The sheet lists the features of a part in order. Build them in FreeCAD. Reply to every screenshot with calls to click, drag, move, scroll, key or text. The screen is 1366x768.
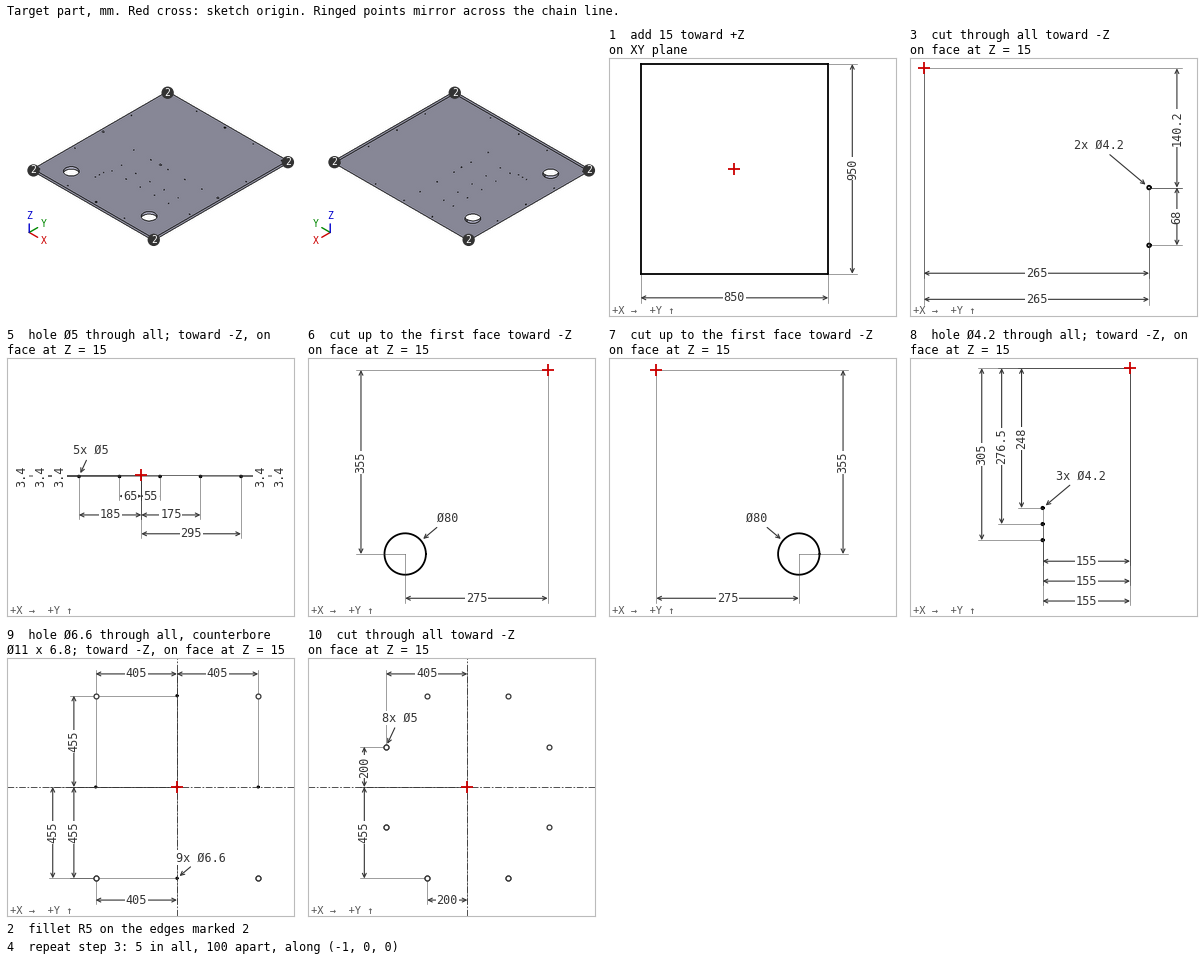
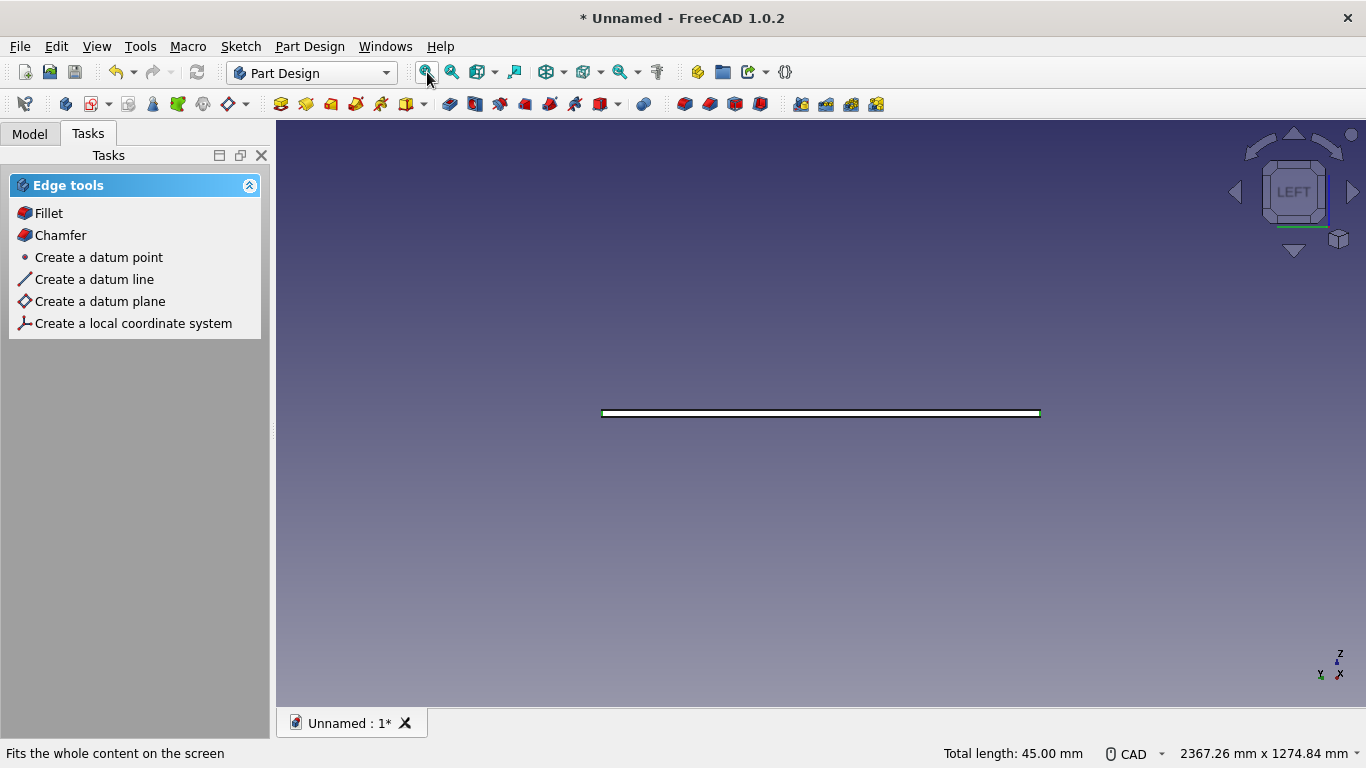
key(0)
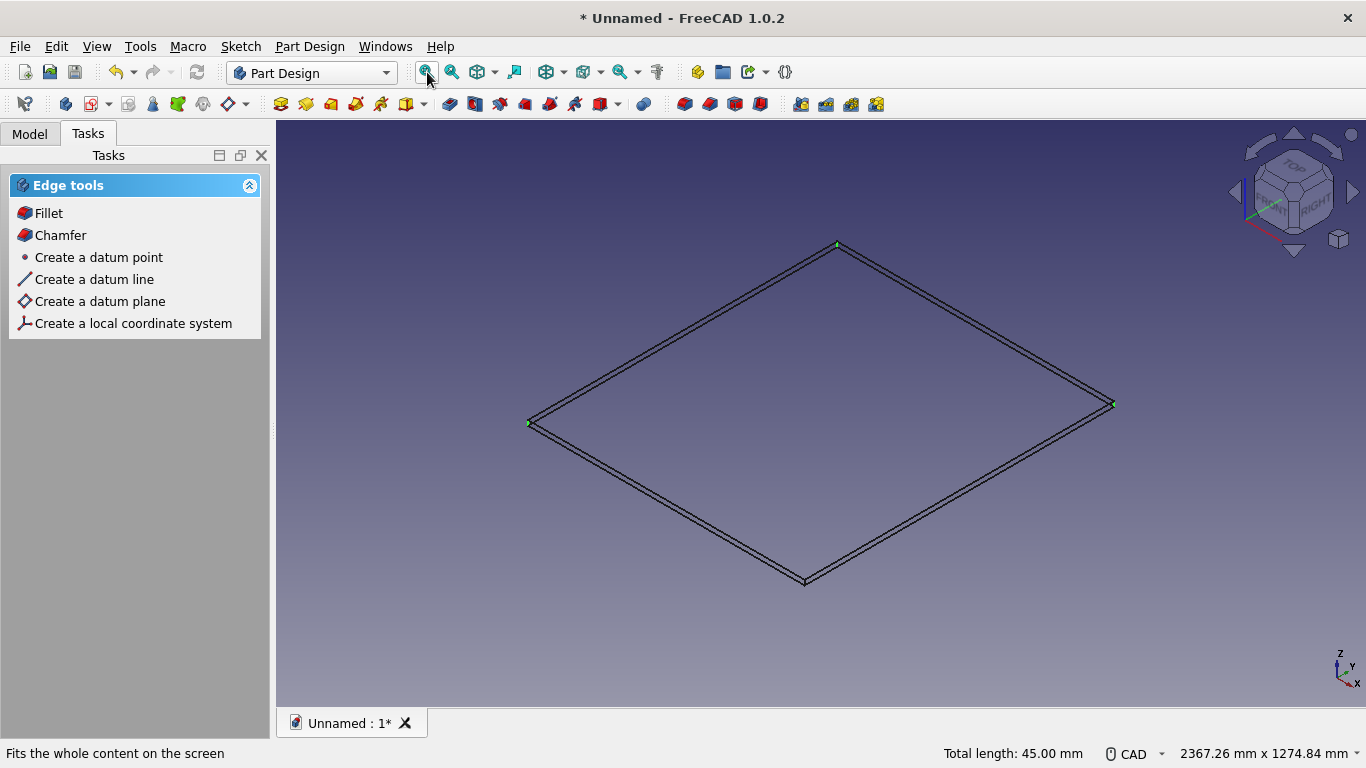
scroll(805, 582, up, 9)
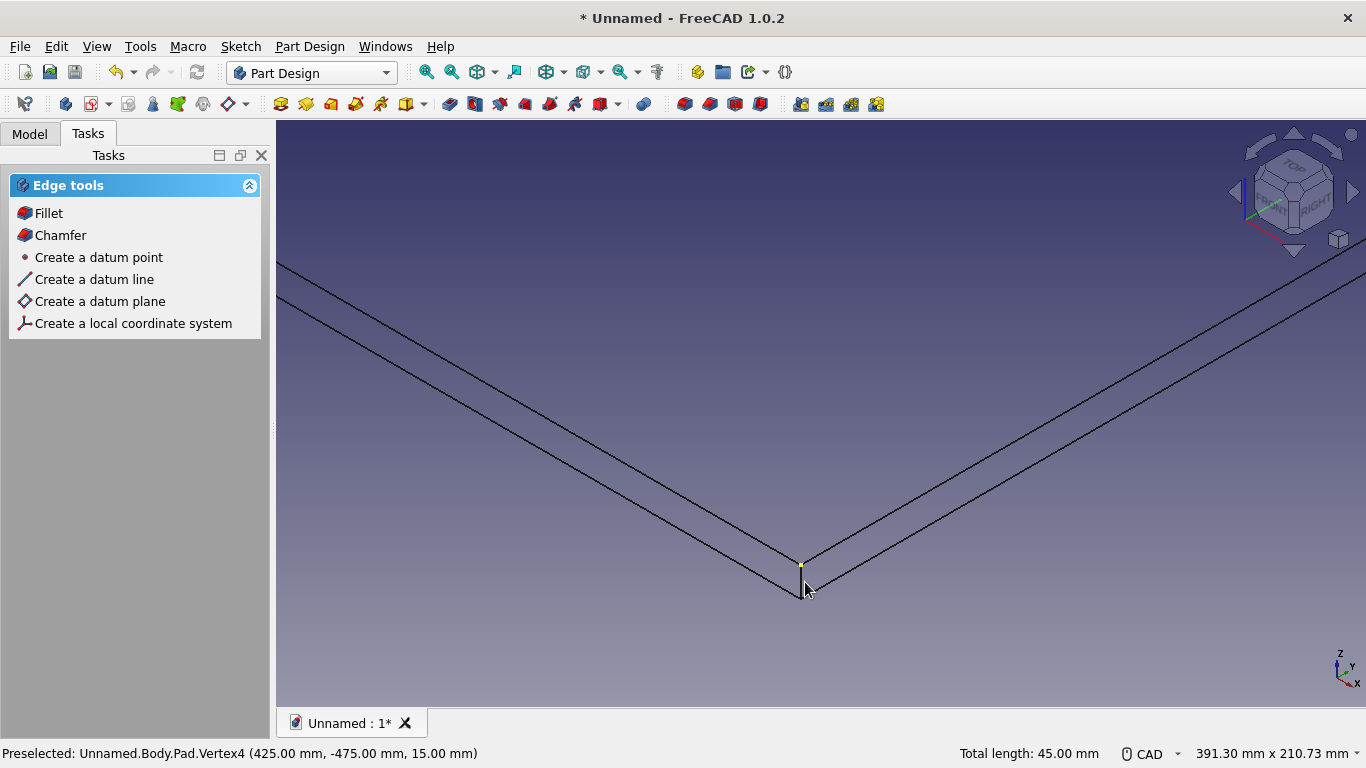
click(801, 581, ctrl)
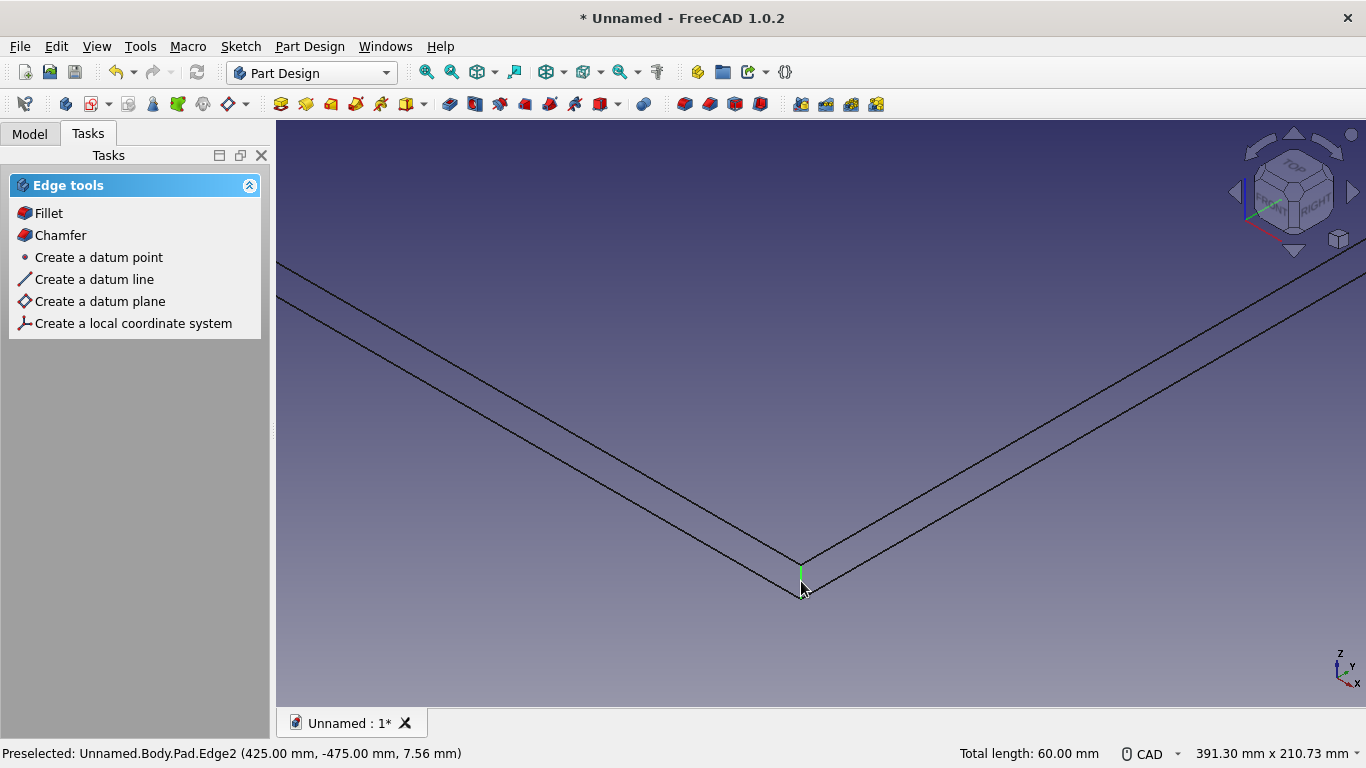
key(v)
key(1)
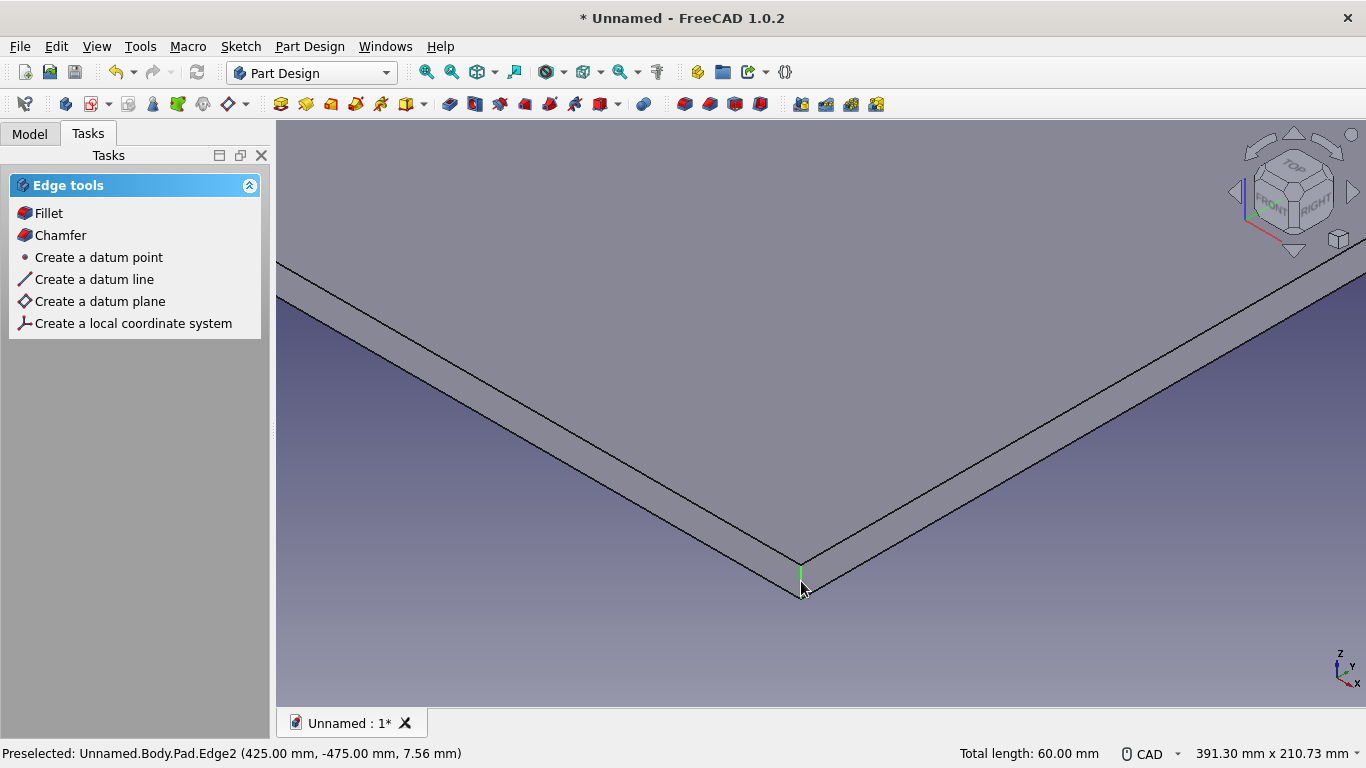
click(685, 104)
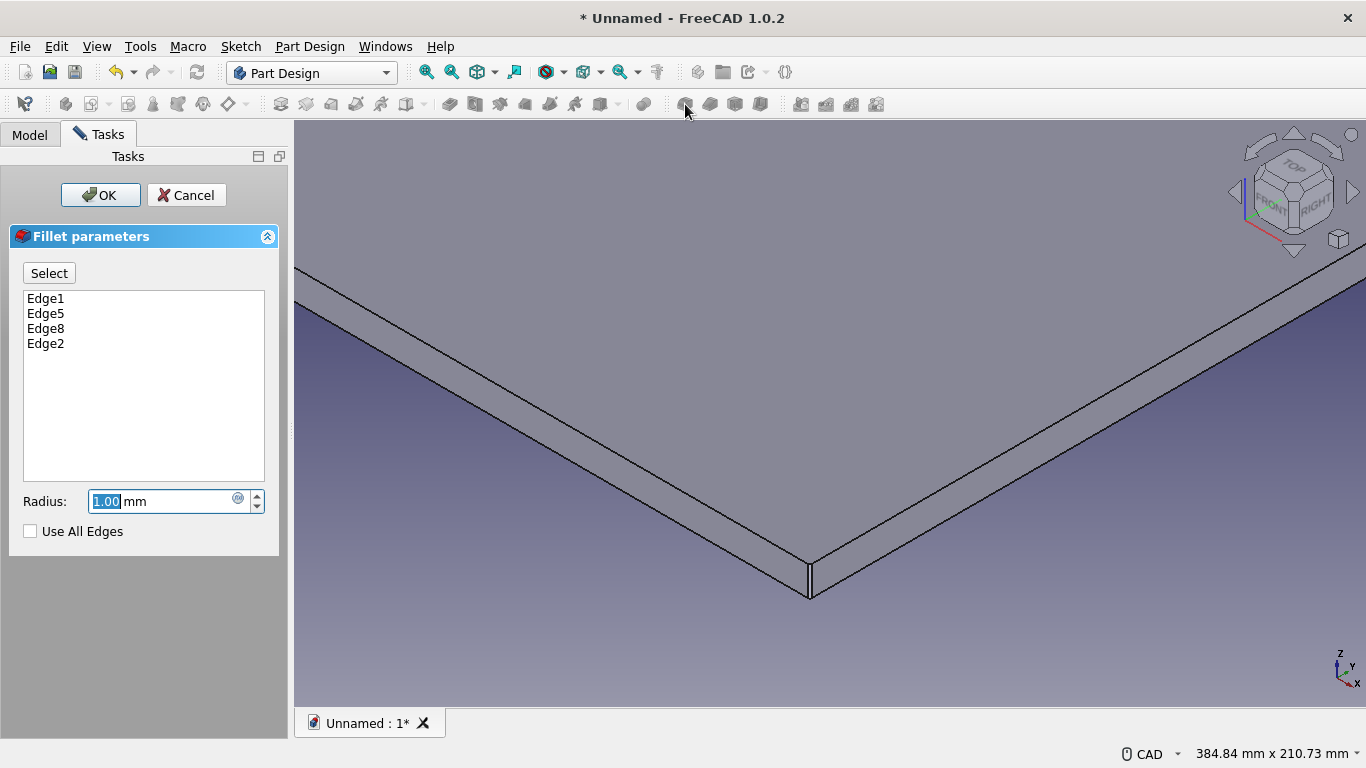
text(5)
key(Tab)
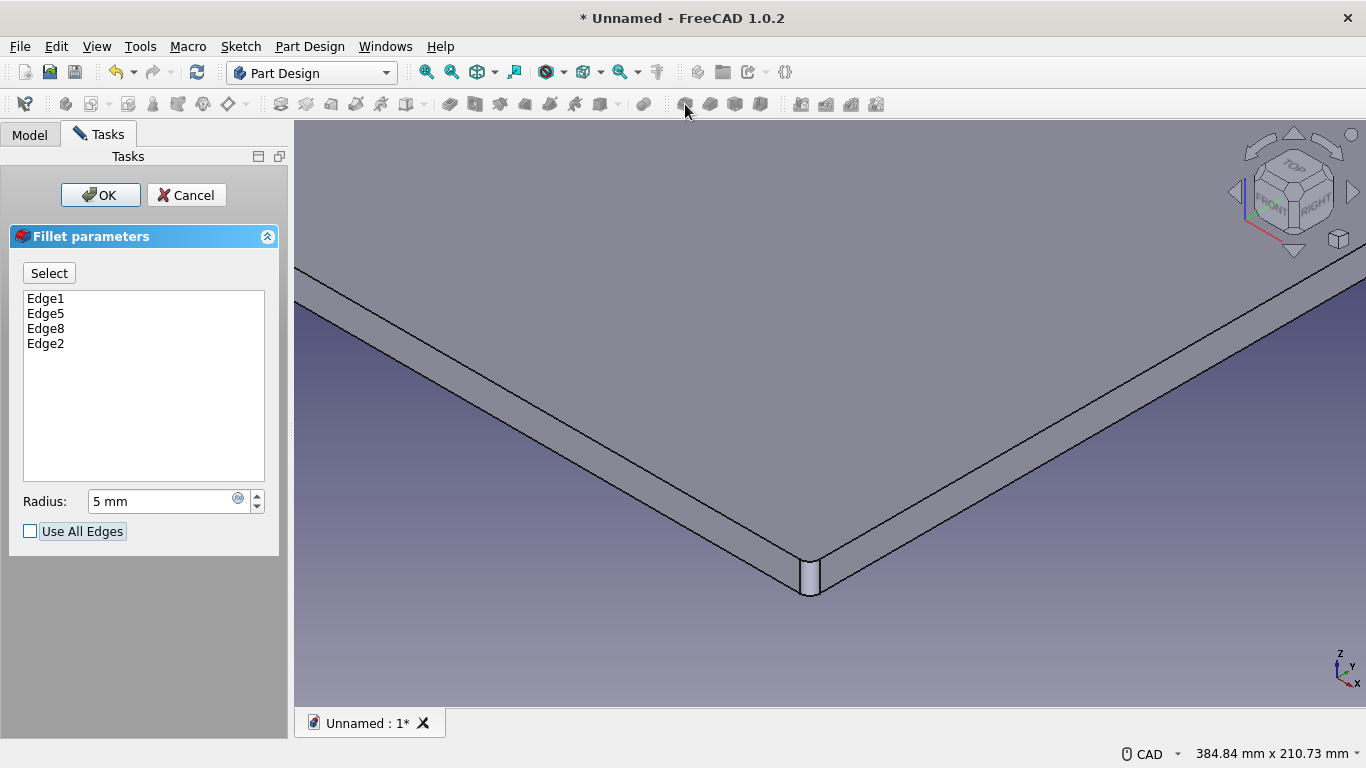
click(101, 195)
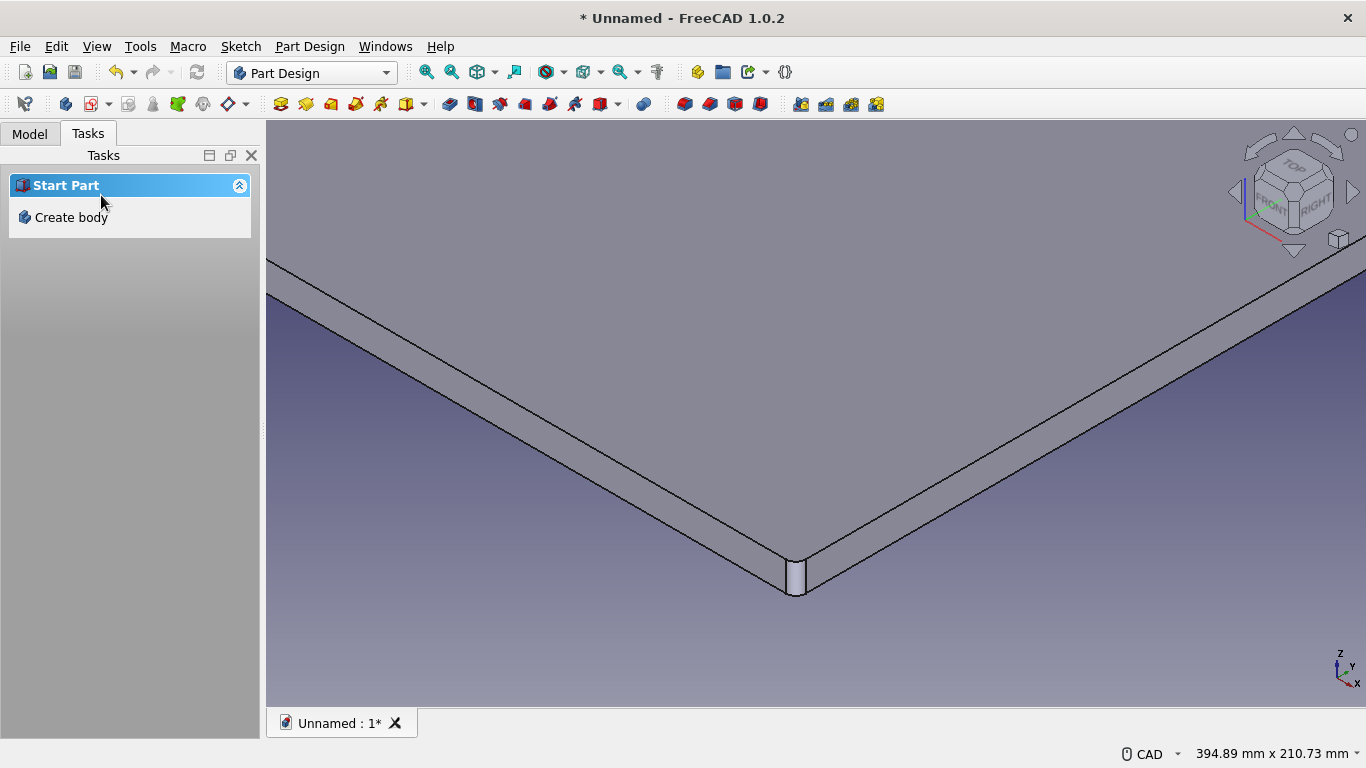
click(427, 72)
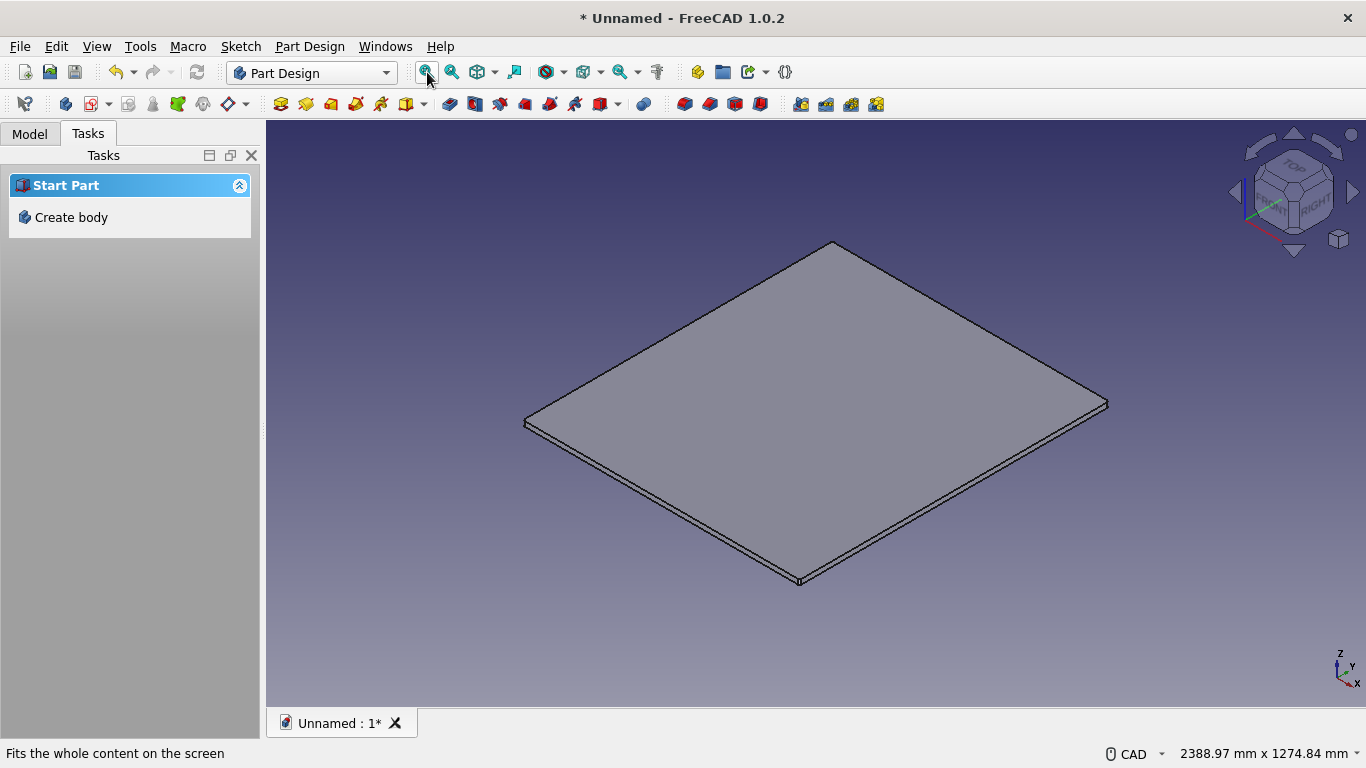
click(816, 410)